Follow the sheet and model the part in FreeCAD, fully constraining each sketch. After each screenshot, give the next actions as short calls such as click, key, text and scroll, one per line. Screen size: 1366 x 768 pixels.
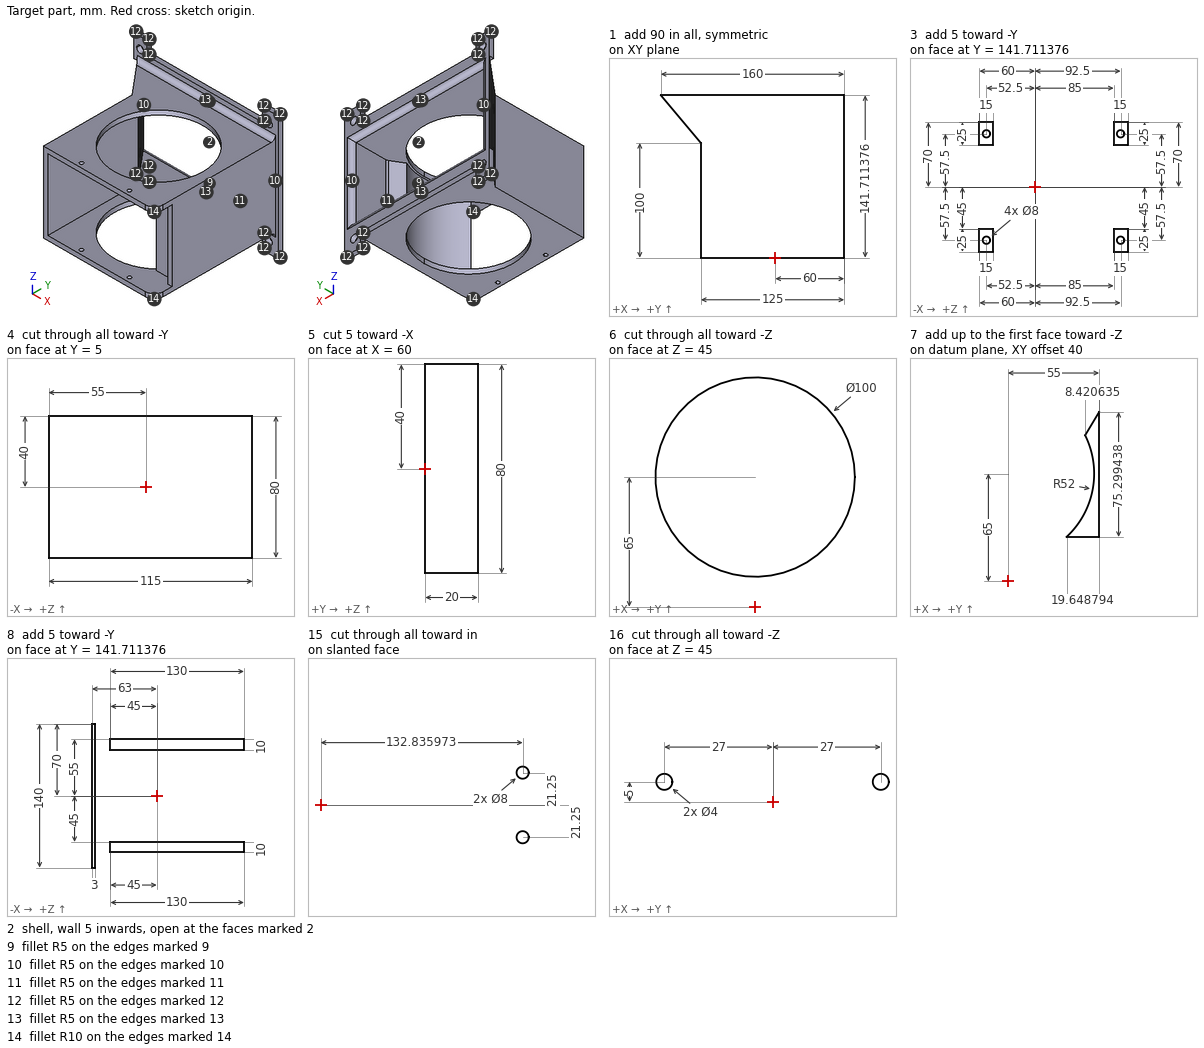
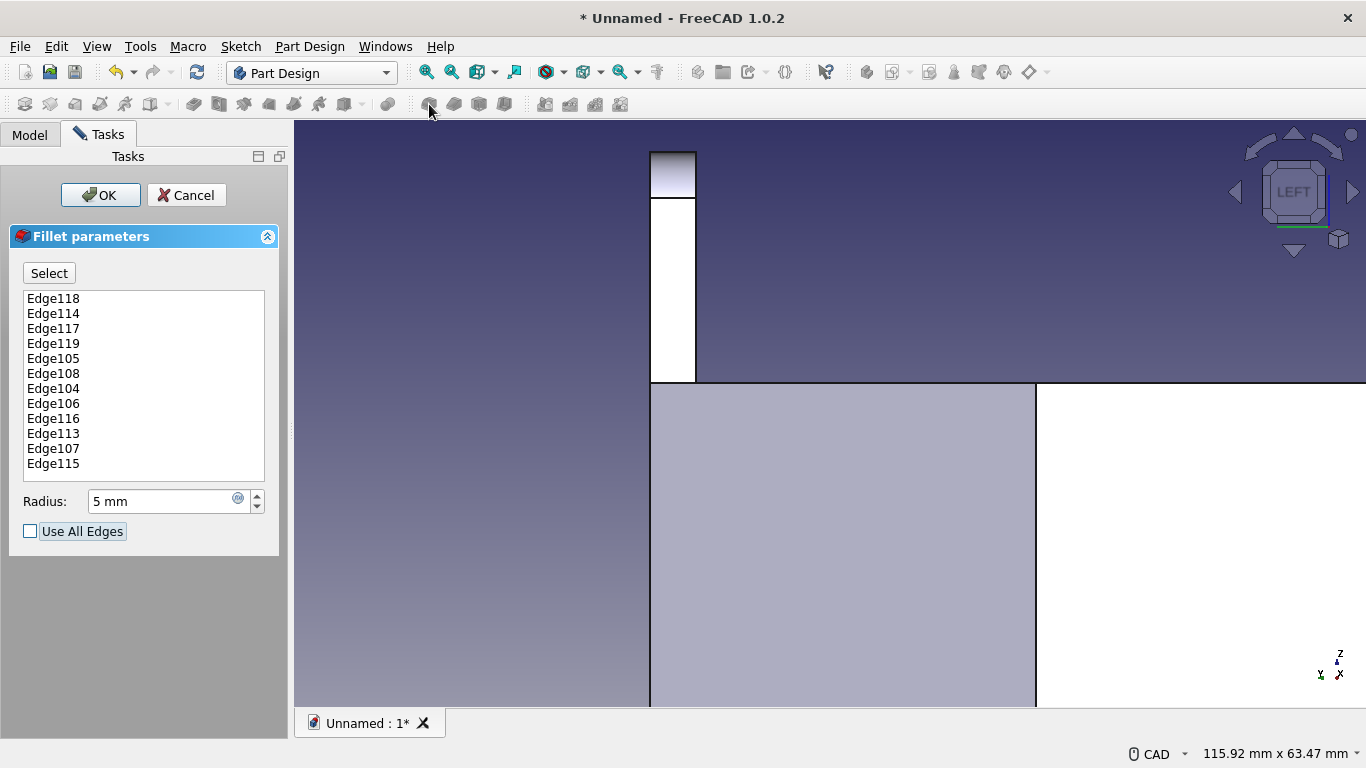
click(101, 195)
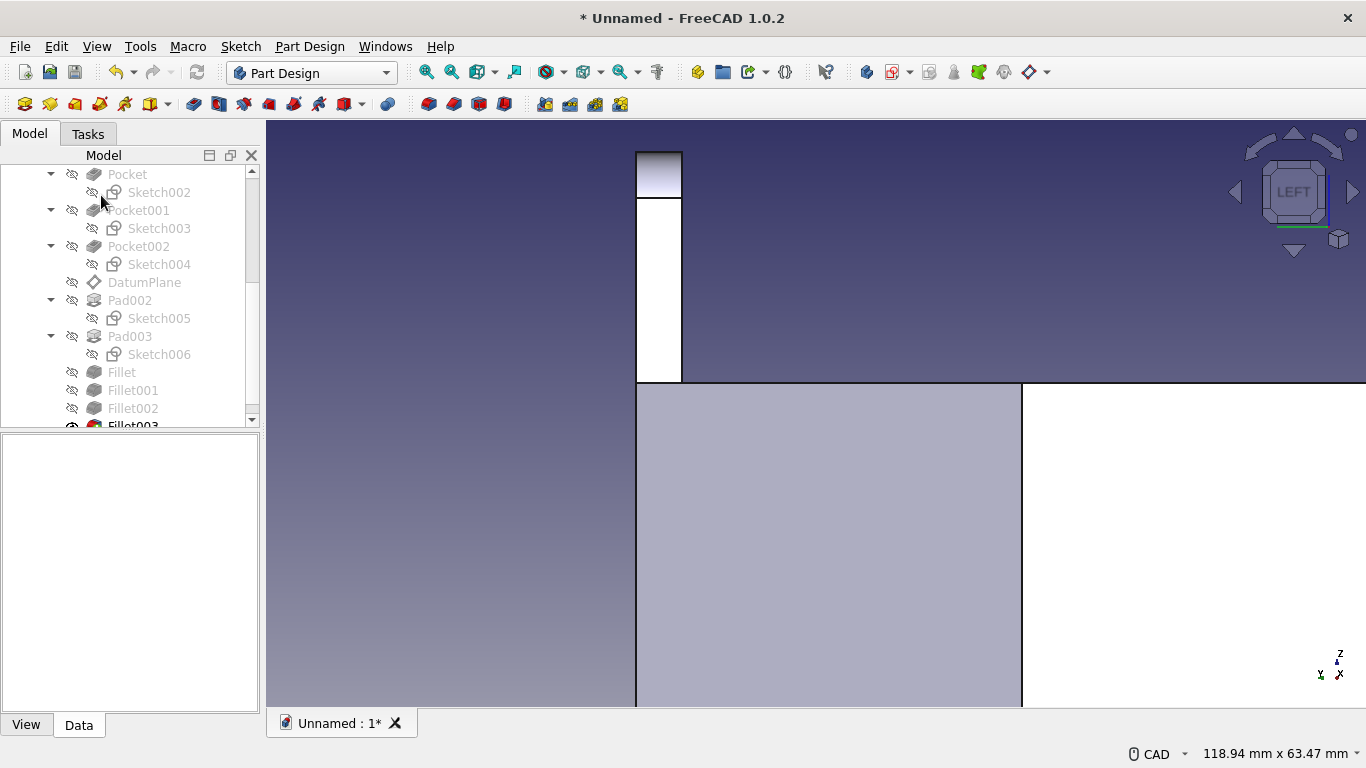
click(427, 72)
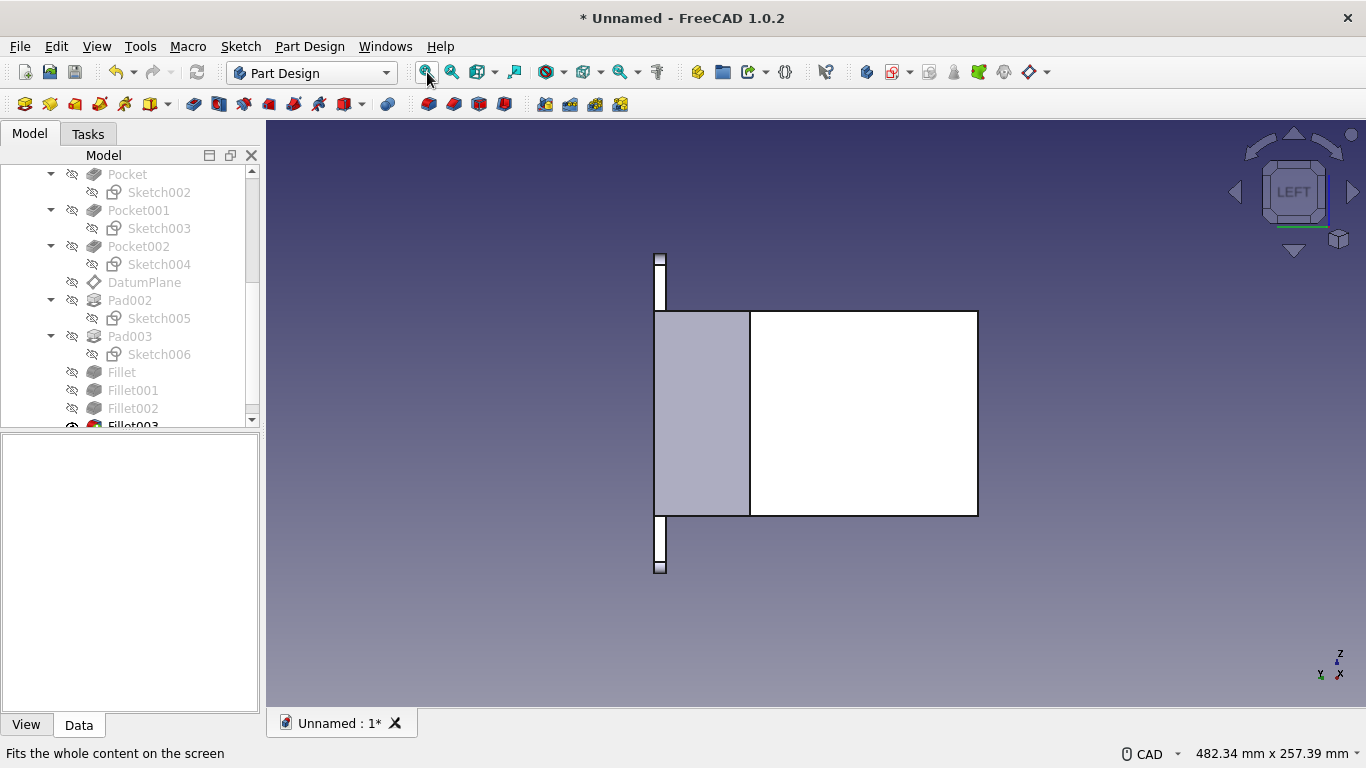
key(0)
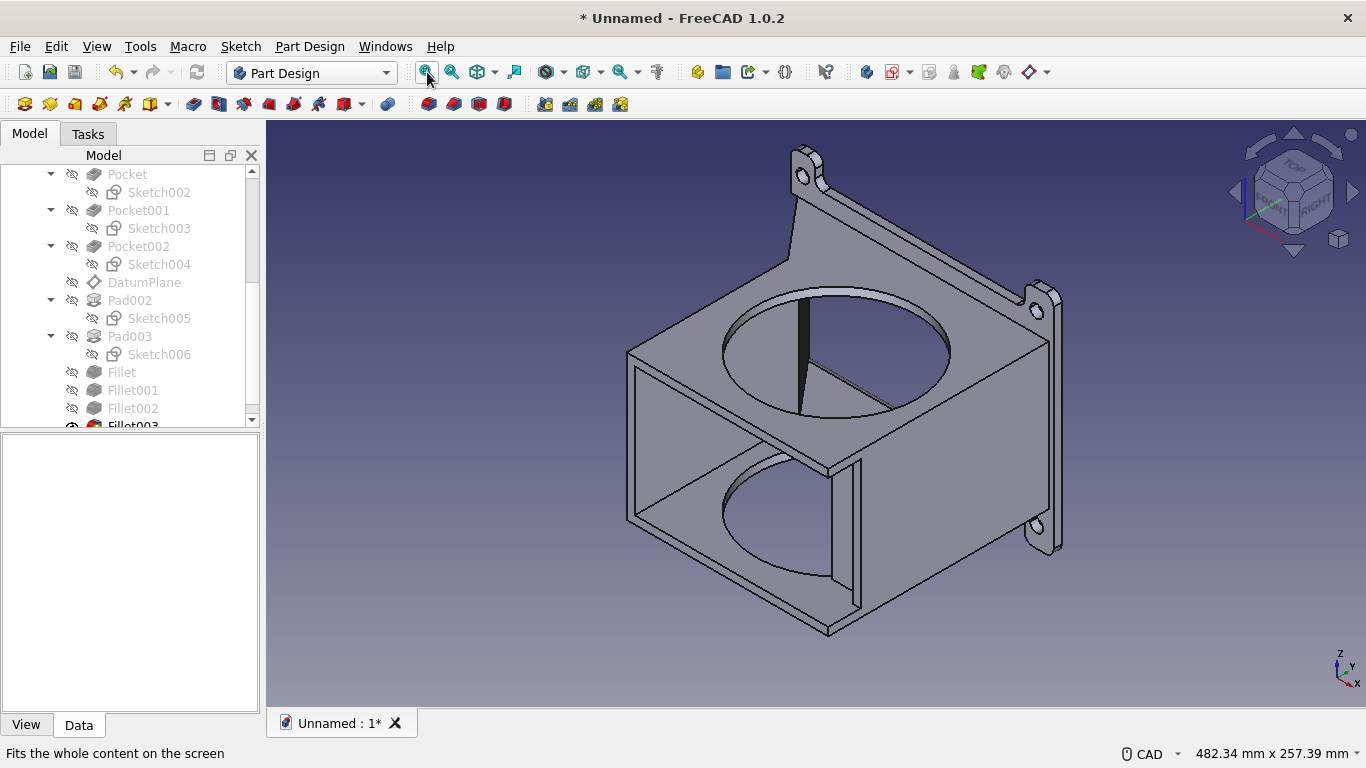
key(2)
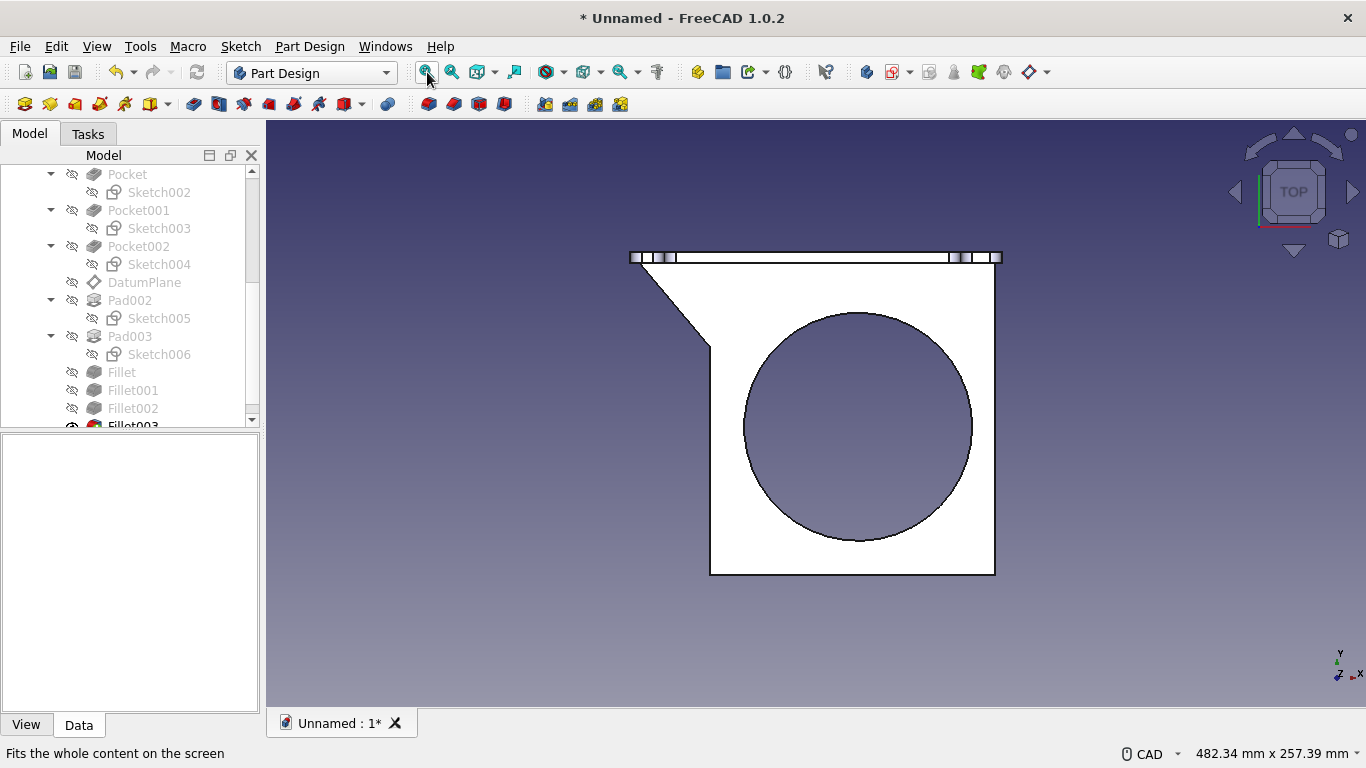
key(1)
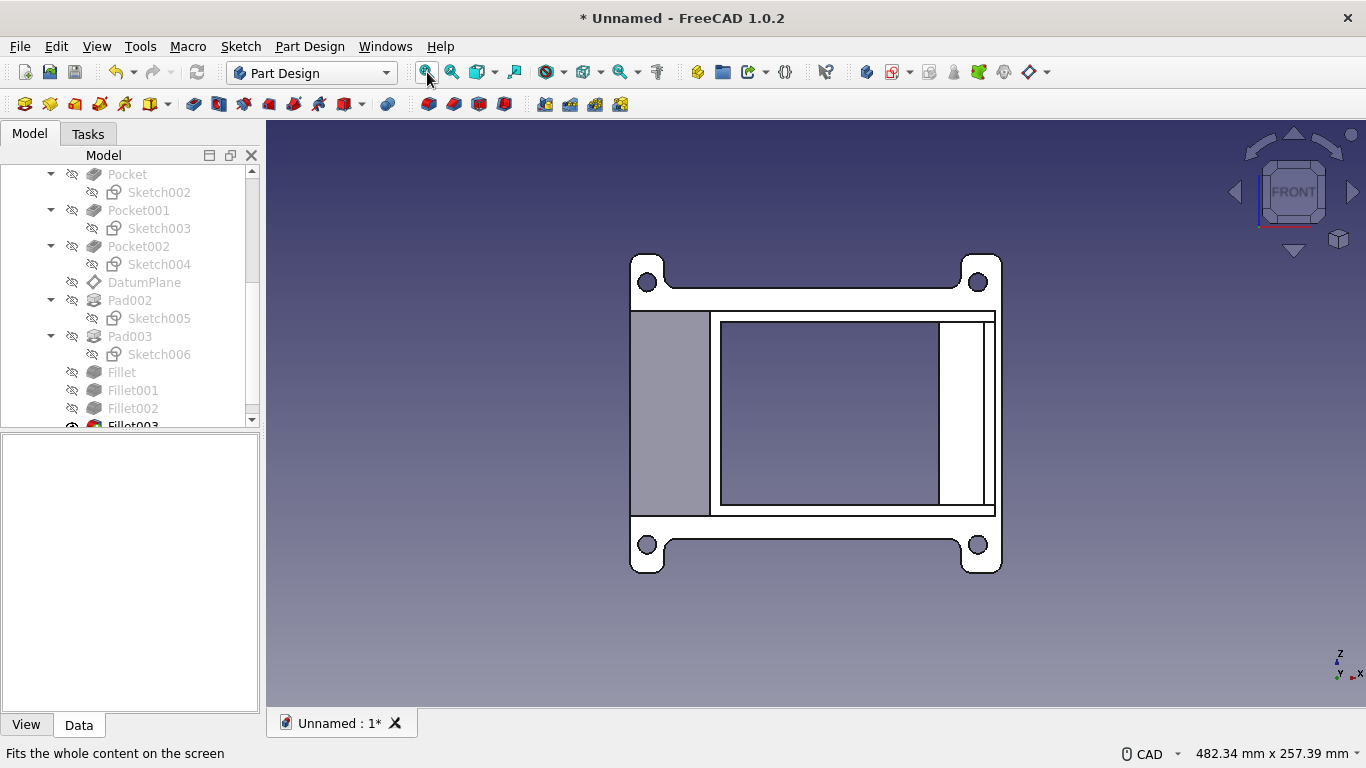
key(3)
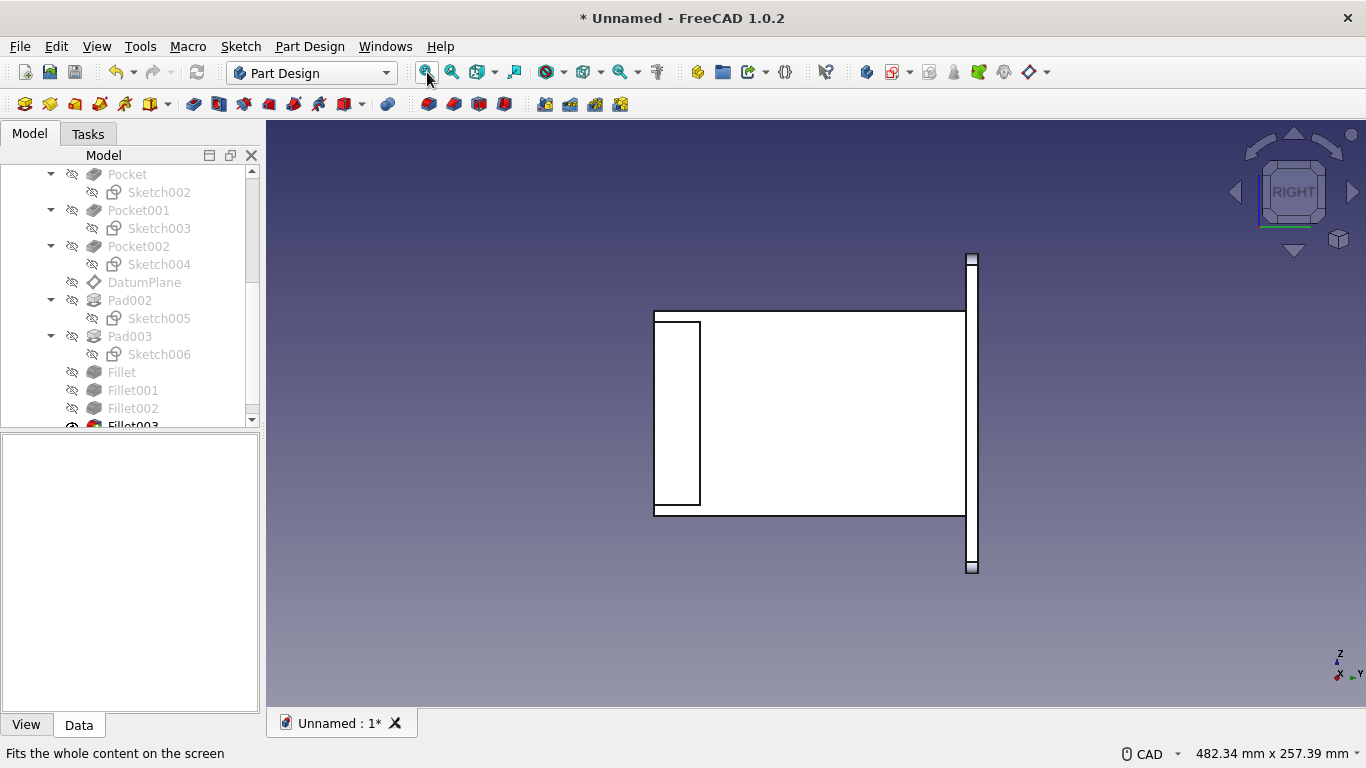
key(5)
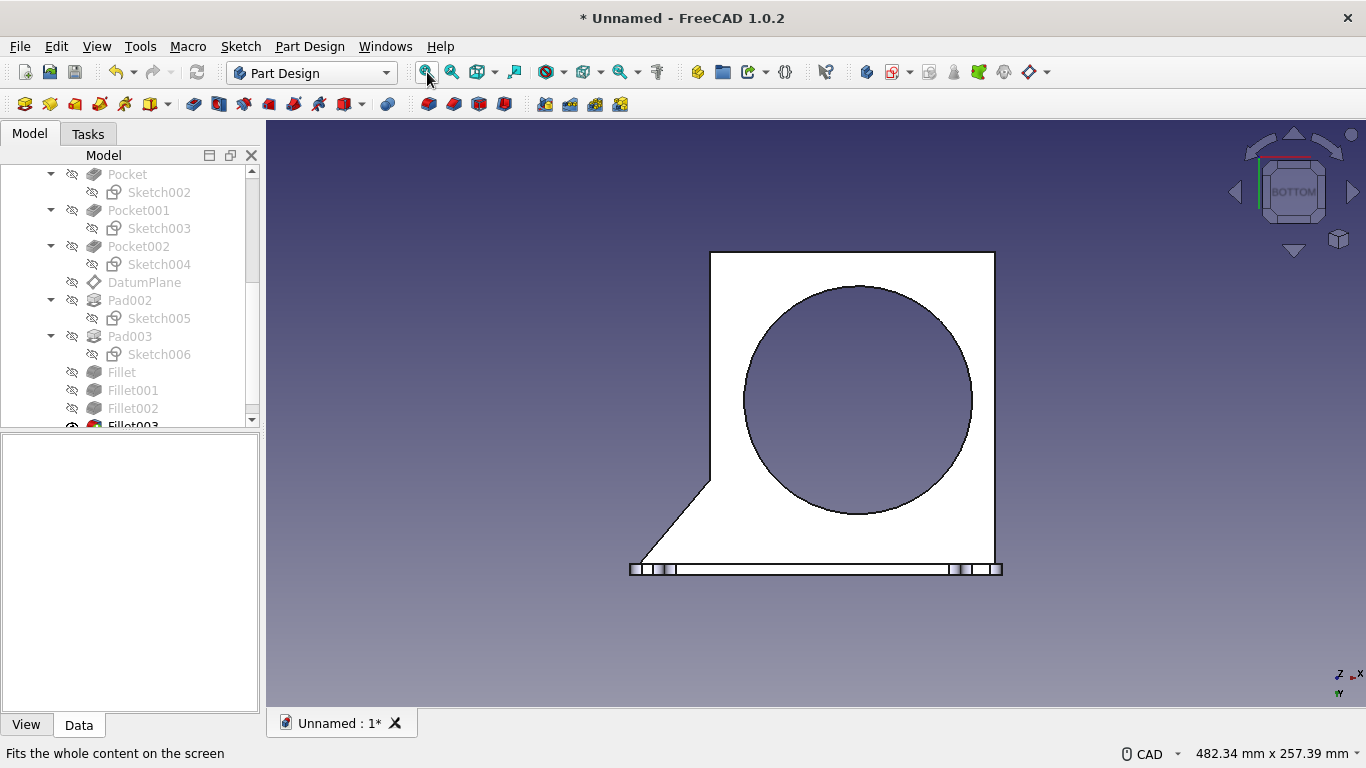
key(4)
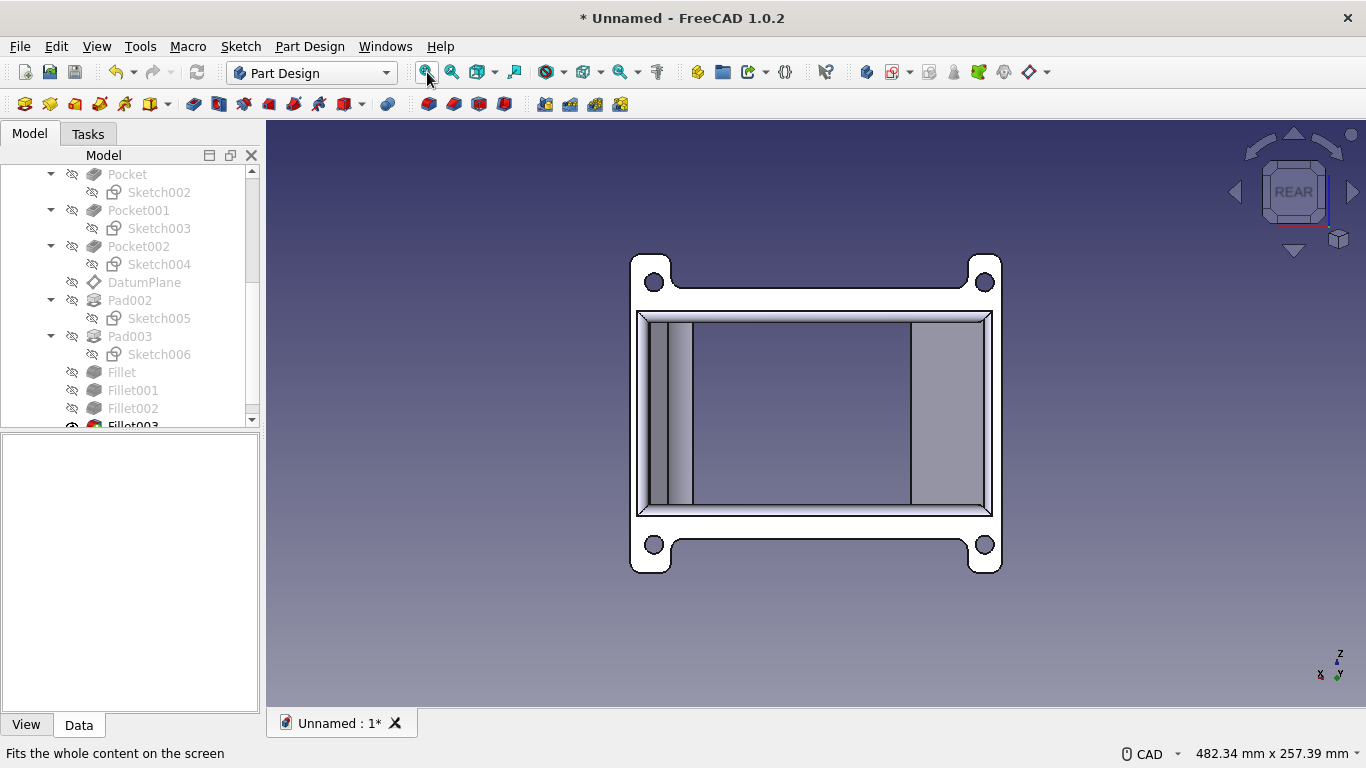
key(6)